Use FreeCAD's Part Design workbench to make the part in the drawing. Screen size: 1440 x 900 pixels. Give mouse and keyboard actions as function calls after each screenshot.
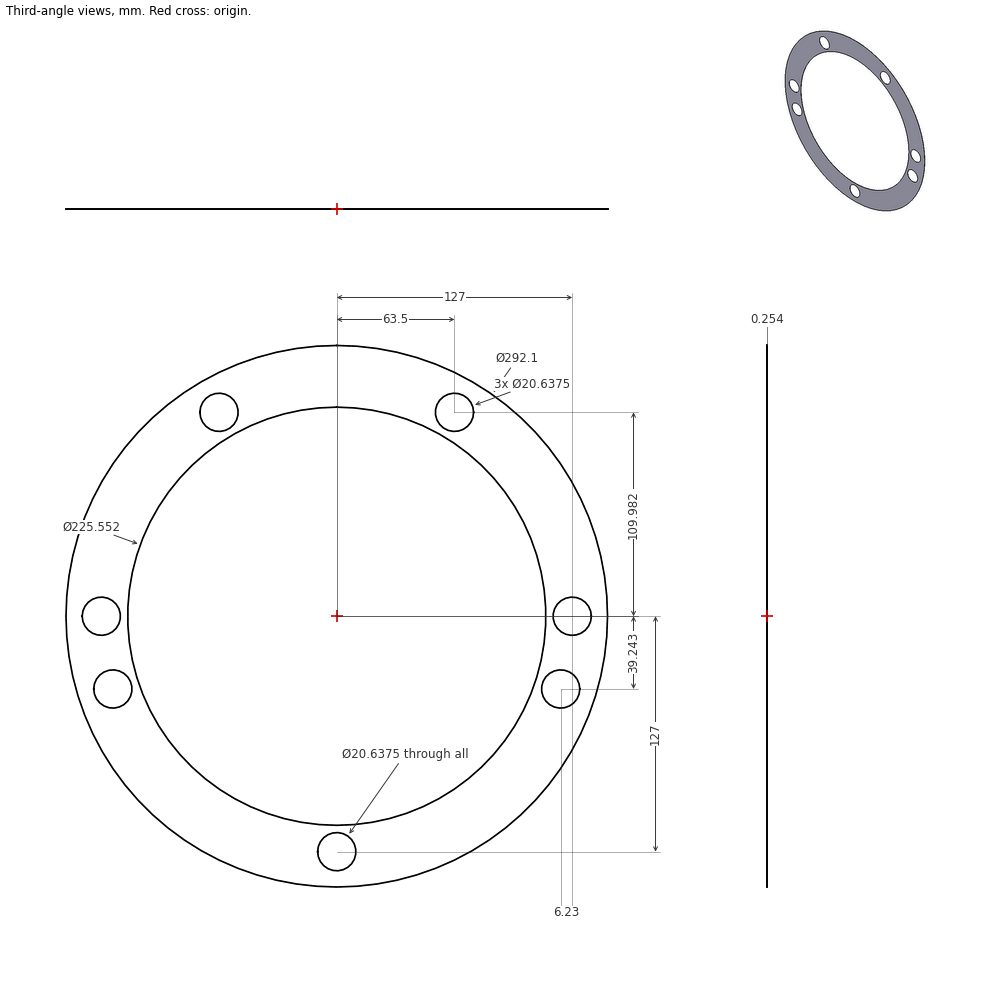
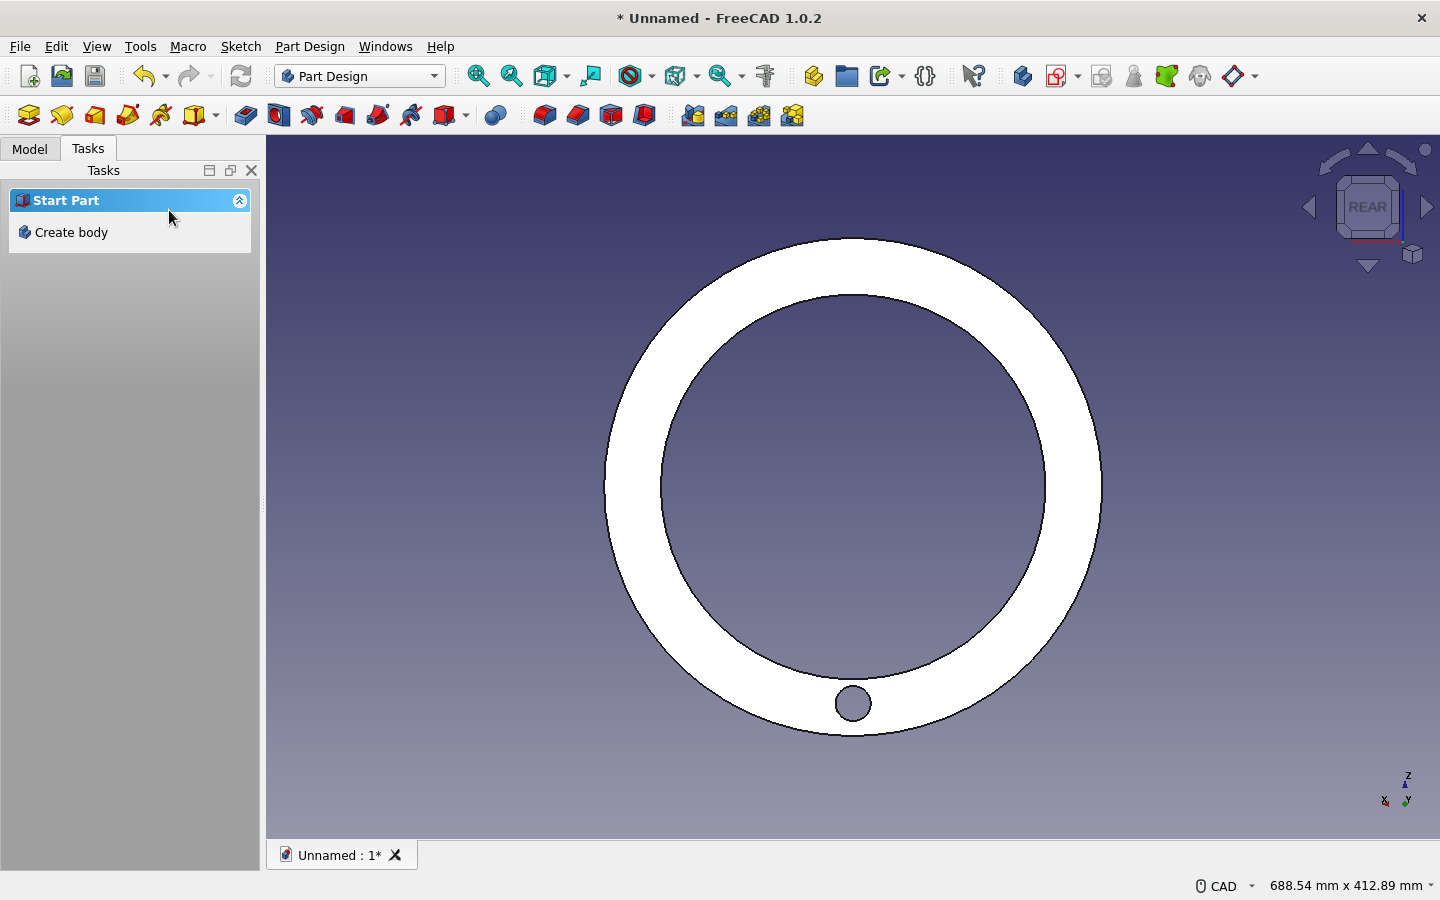
click(1056, 76)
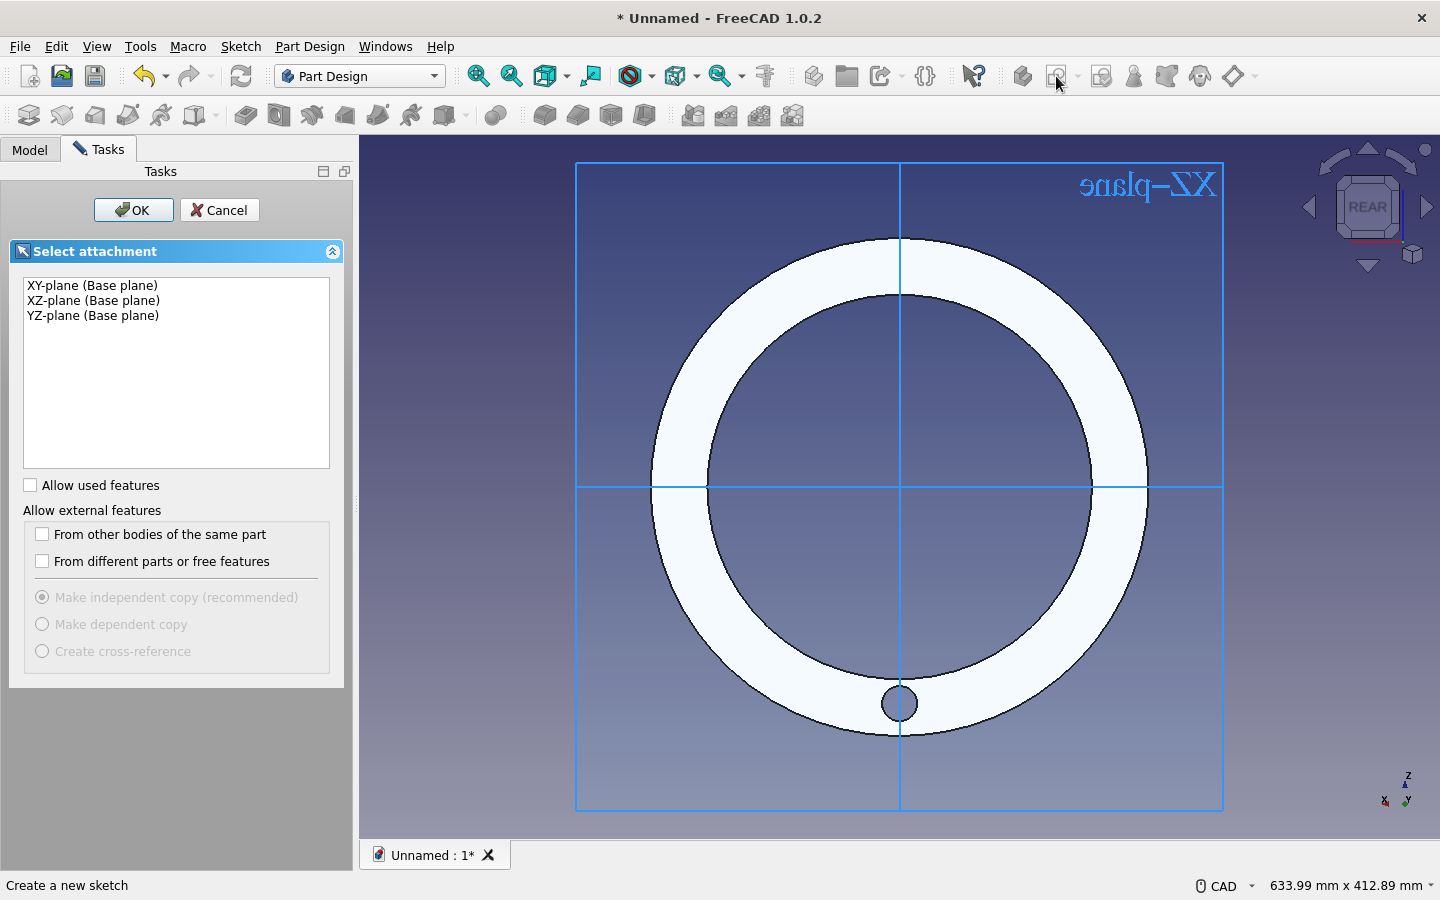
click(84, 300)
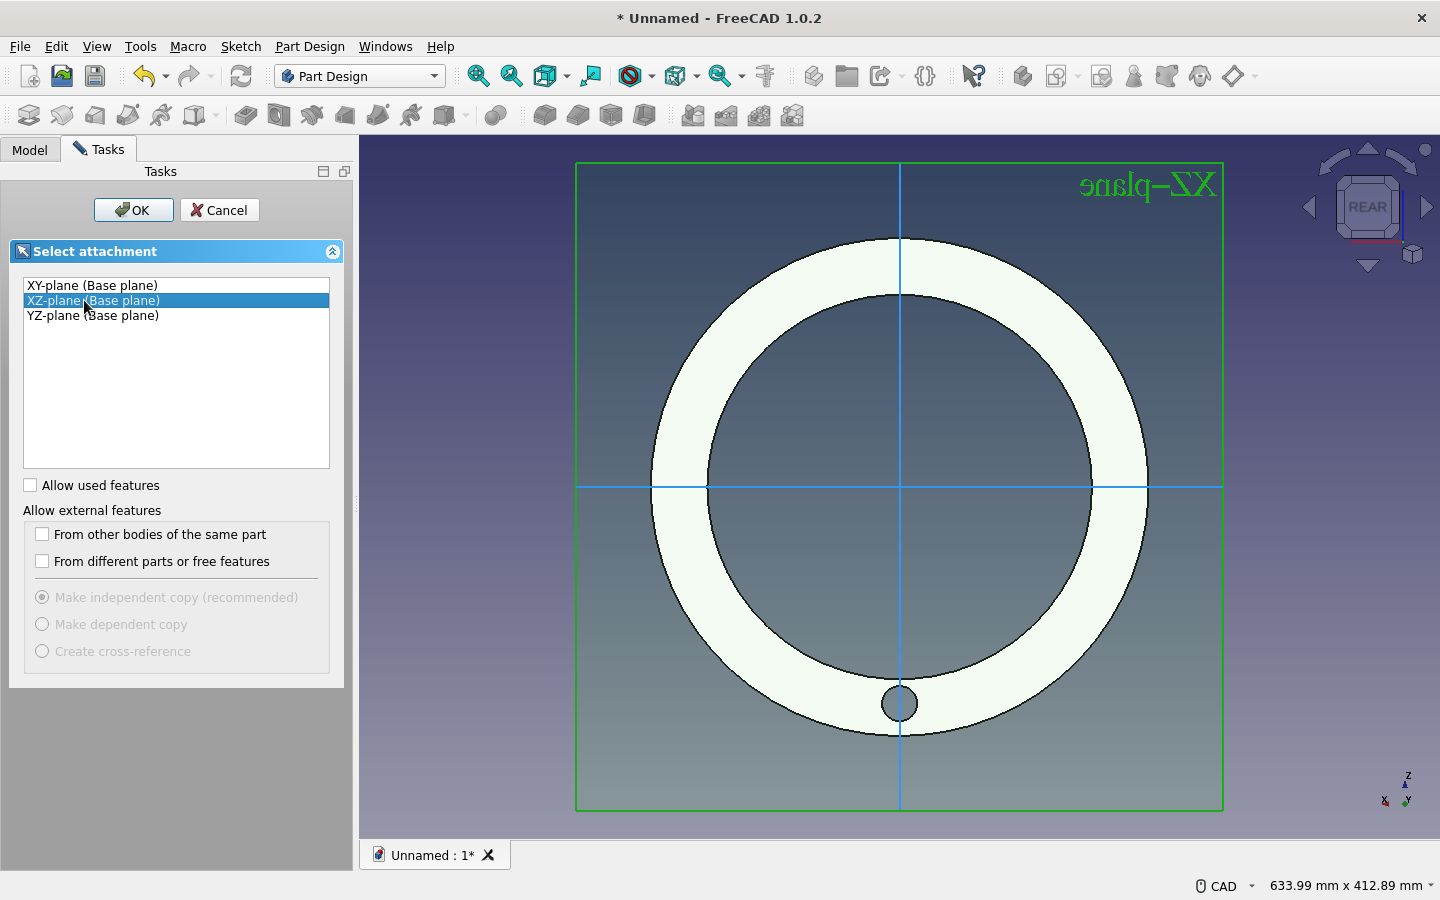
click(134, 210)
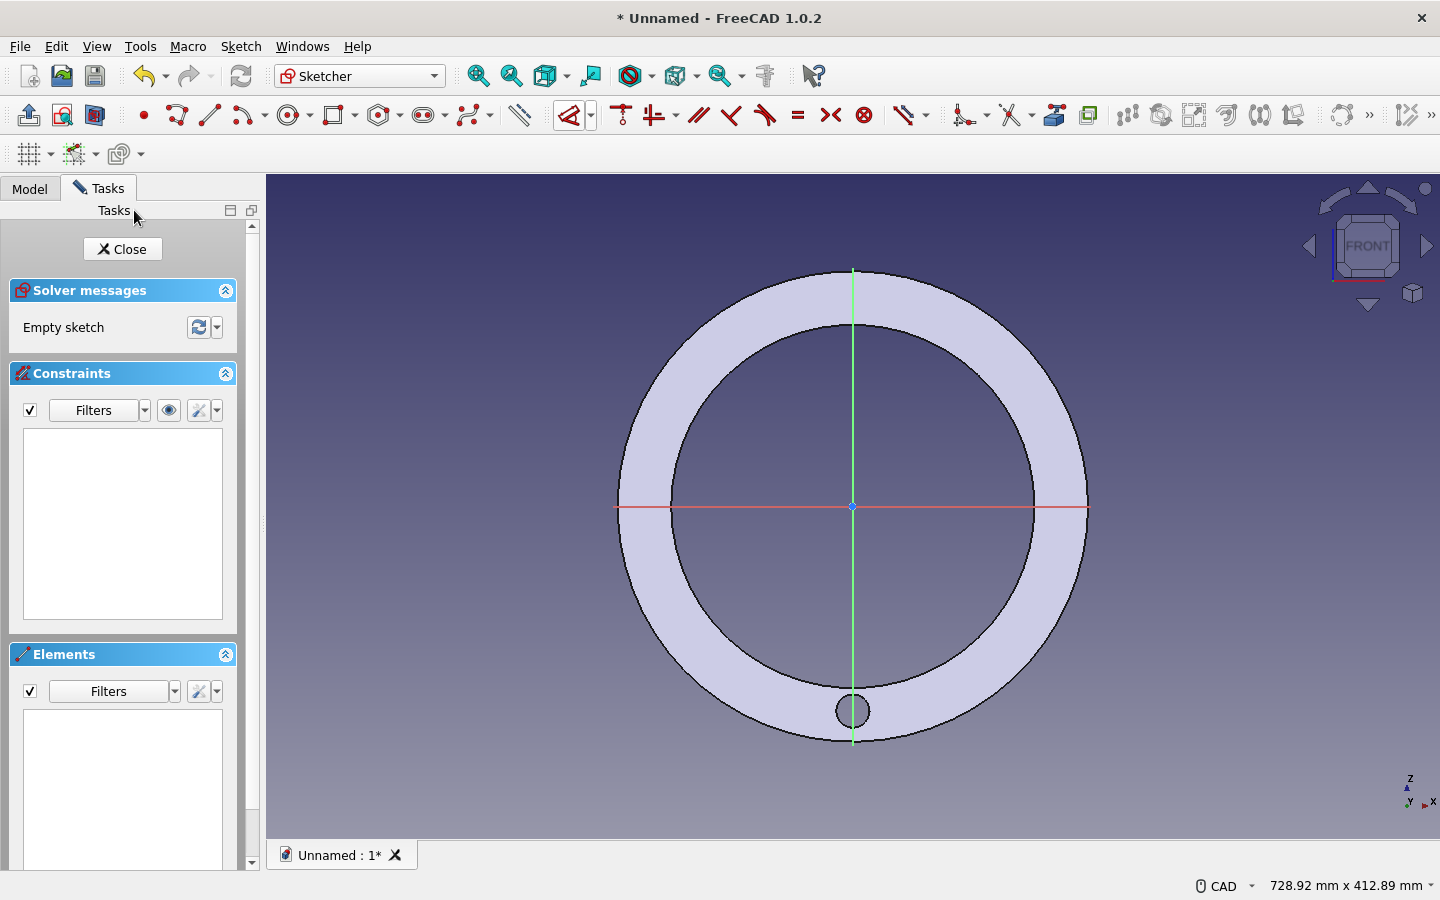
scroll(1275, 334, up, 2)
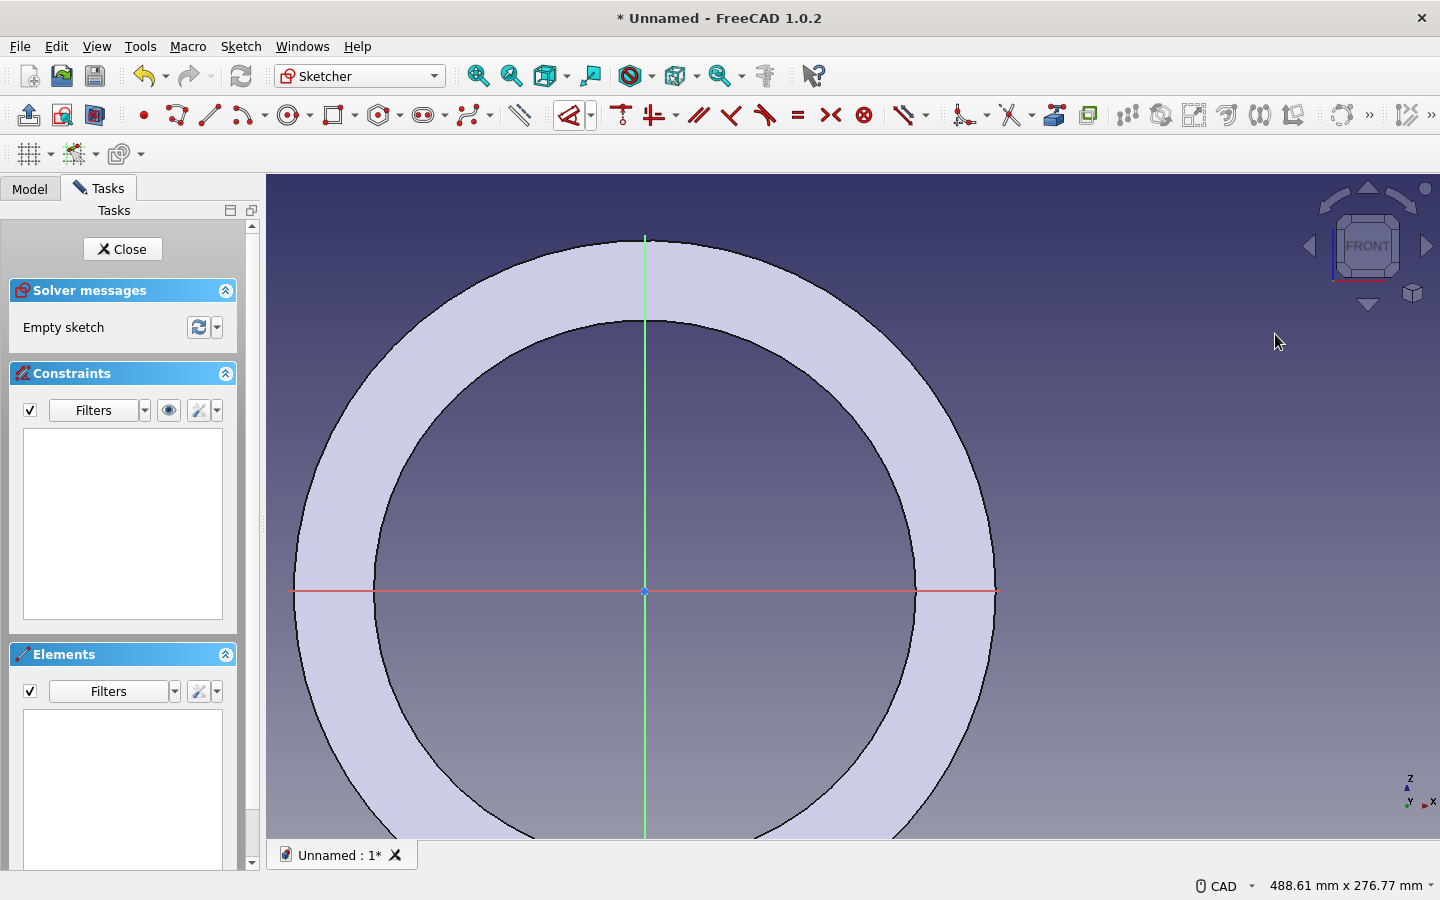
click(288, 116)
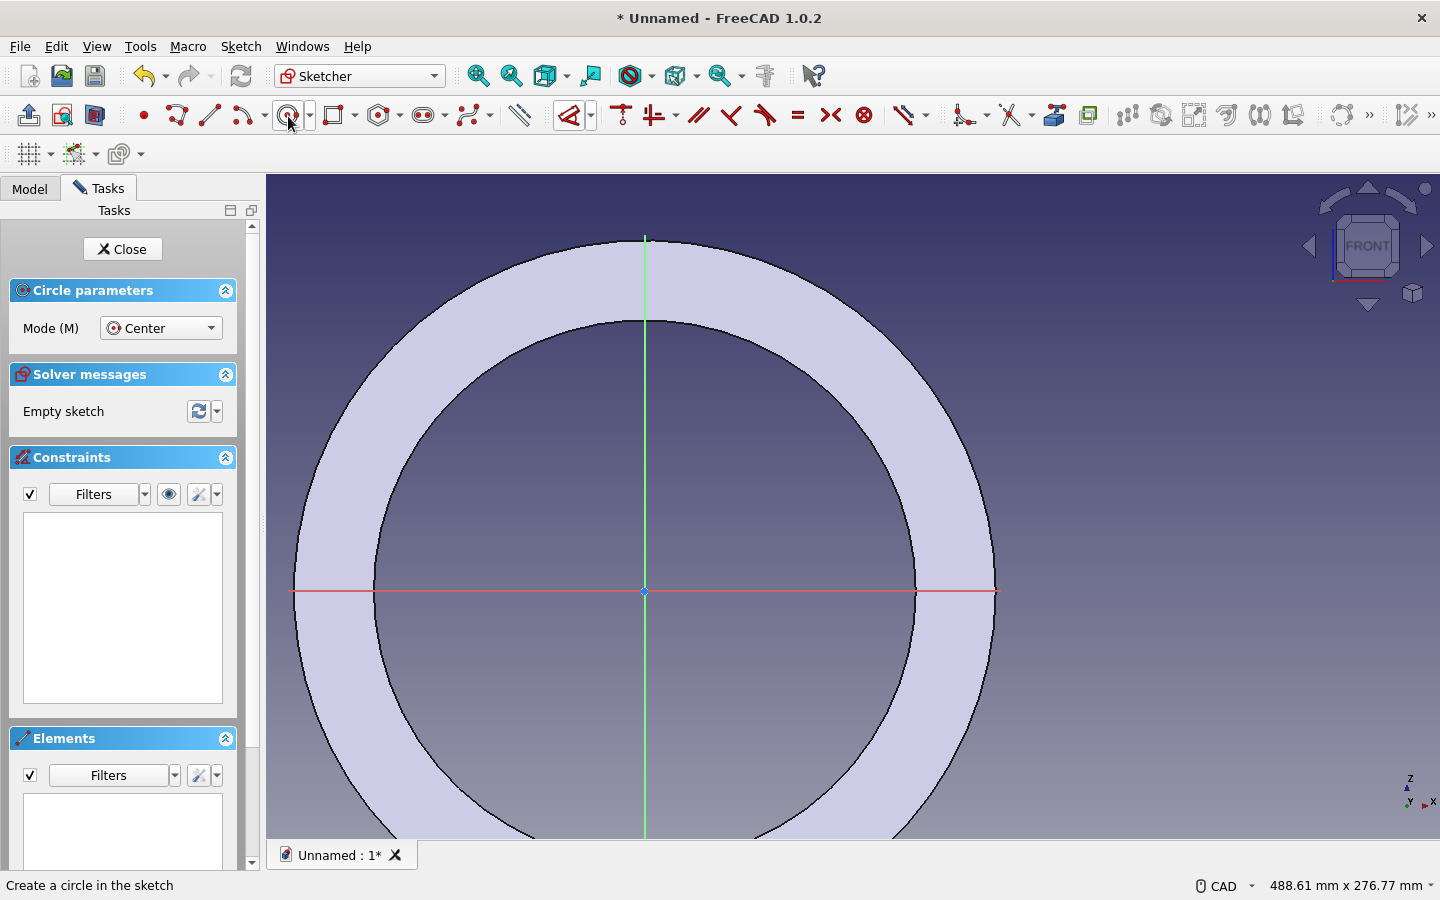
click(797, 327)
click(815, 309)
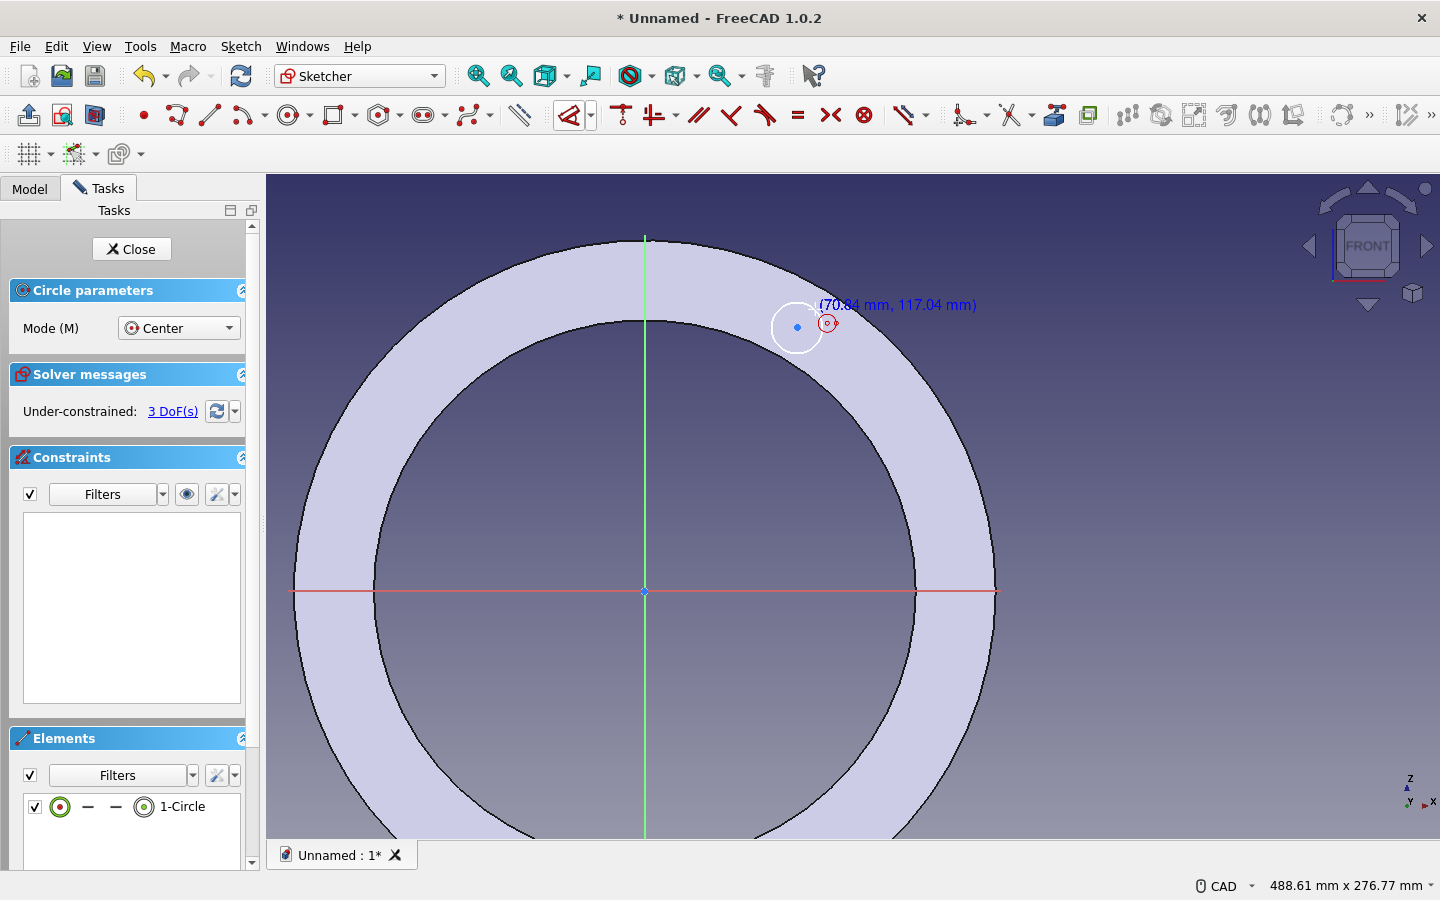
click(935, 686)
click(953, 668)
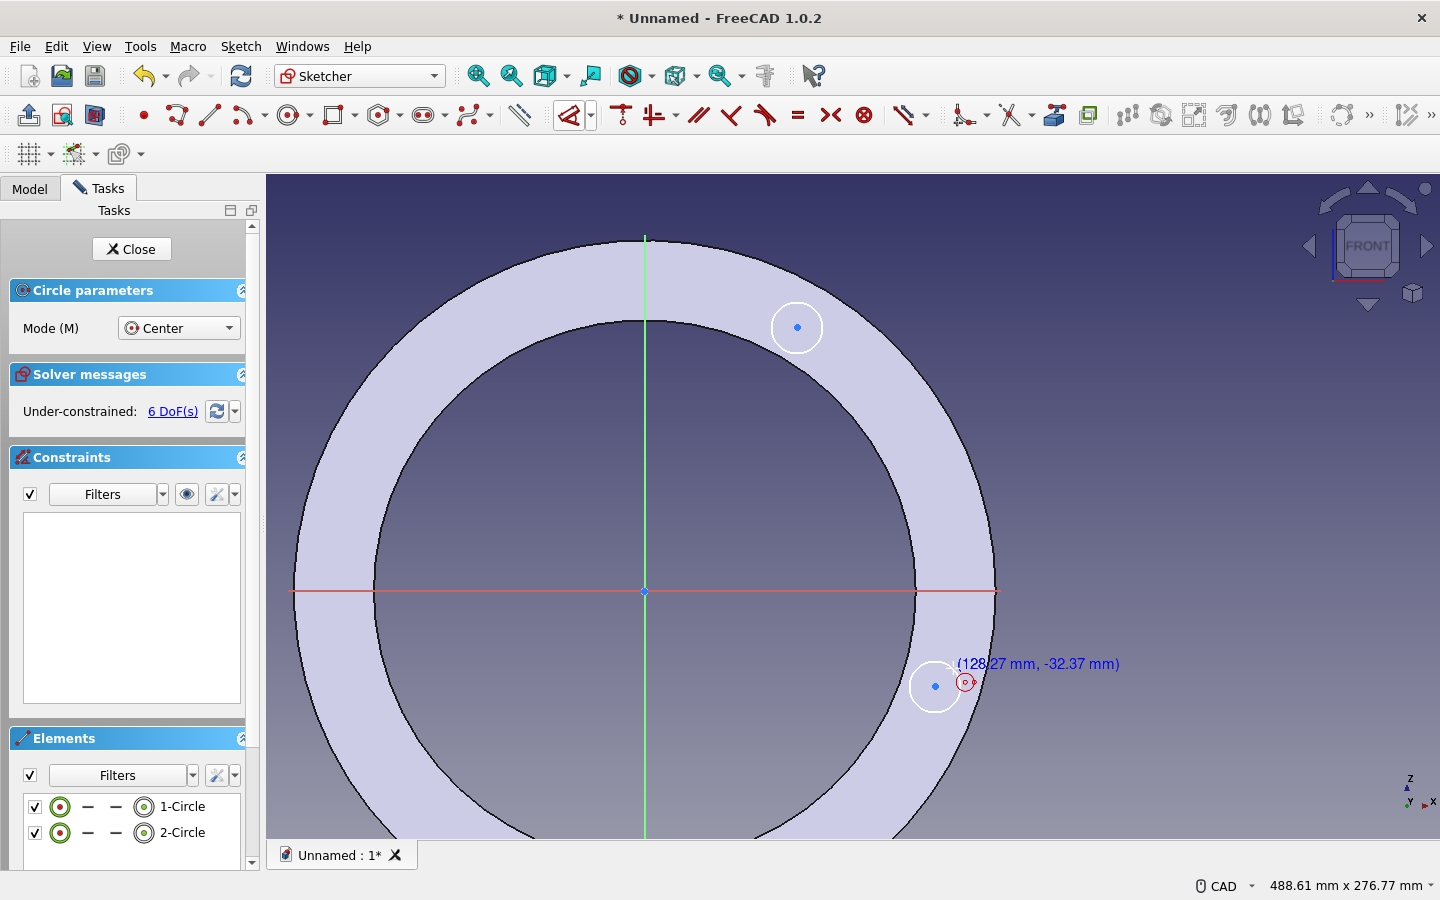
click(950, 591)
click(967, 574)
key(Escape)